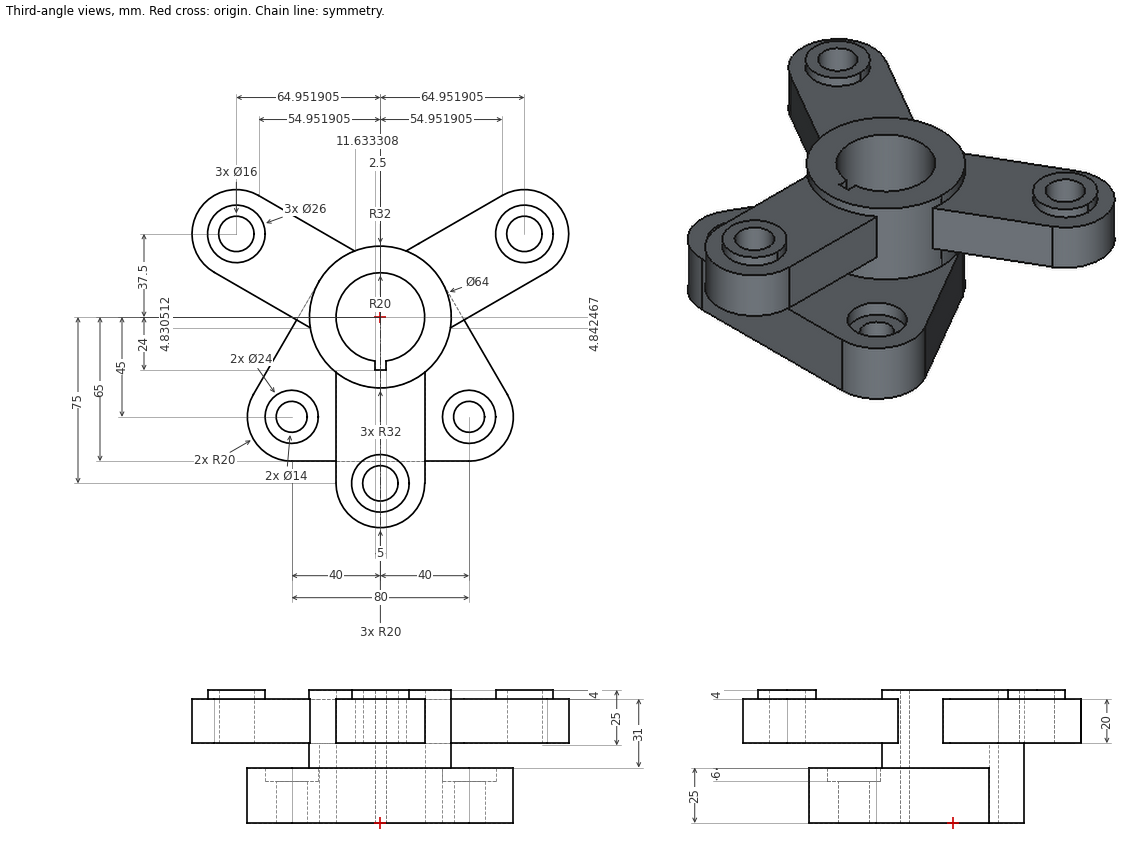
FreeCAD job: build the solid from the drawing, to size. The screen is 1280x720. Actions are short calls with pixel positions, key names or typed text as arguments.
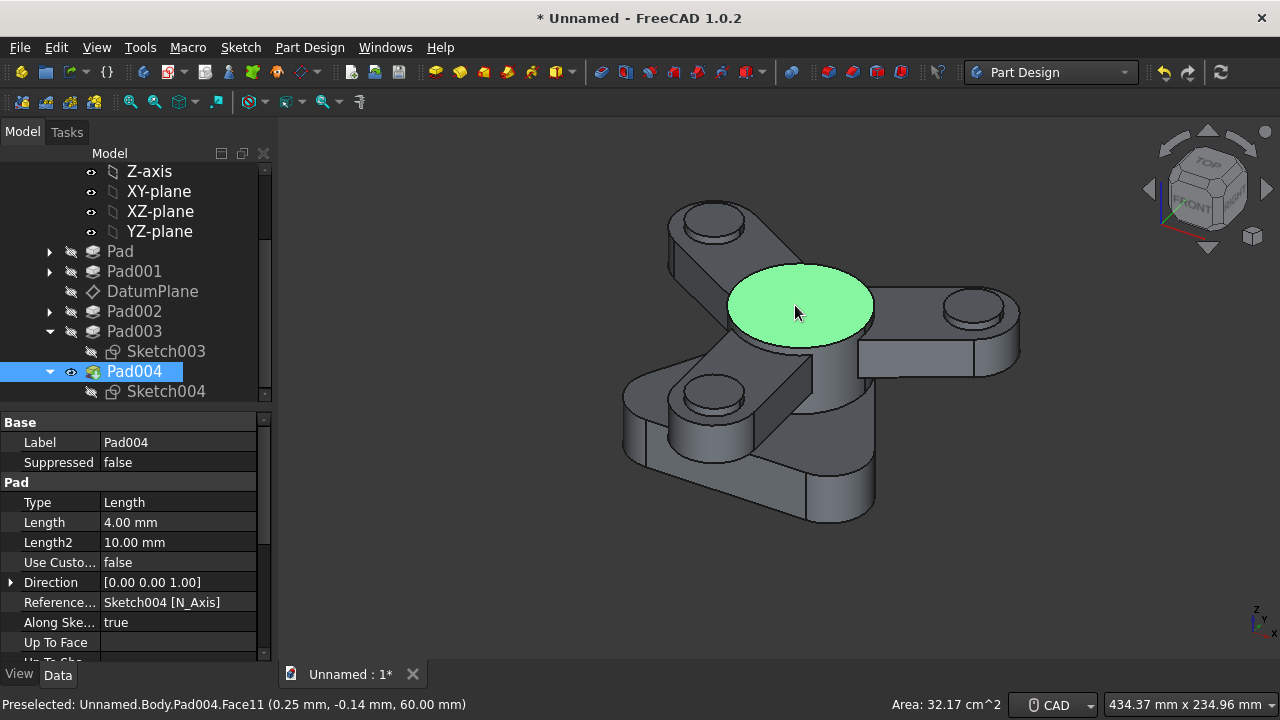
click(168, 72)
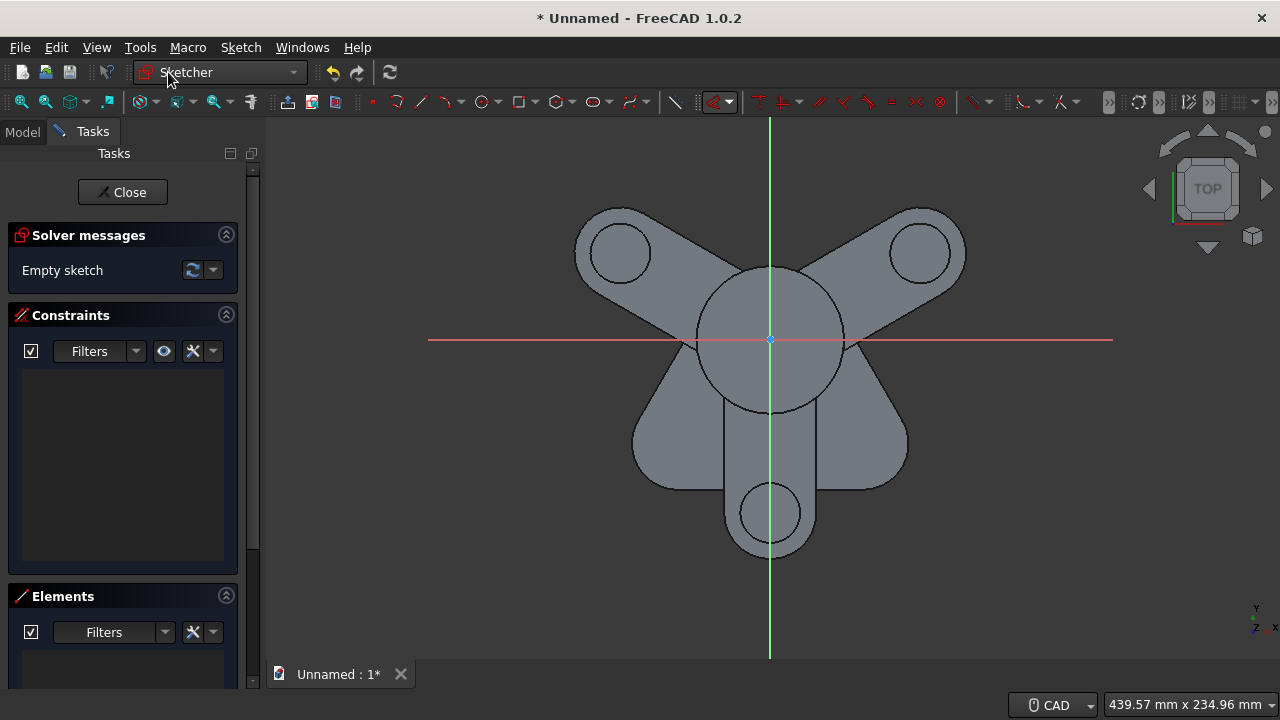
key(g)
key(c)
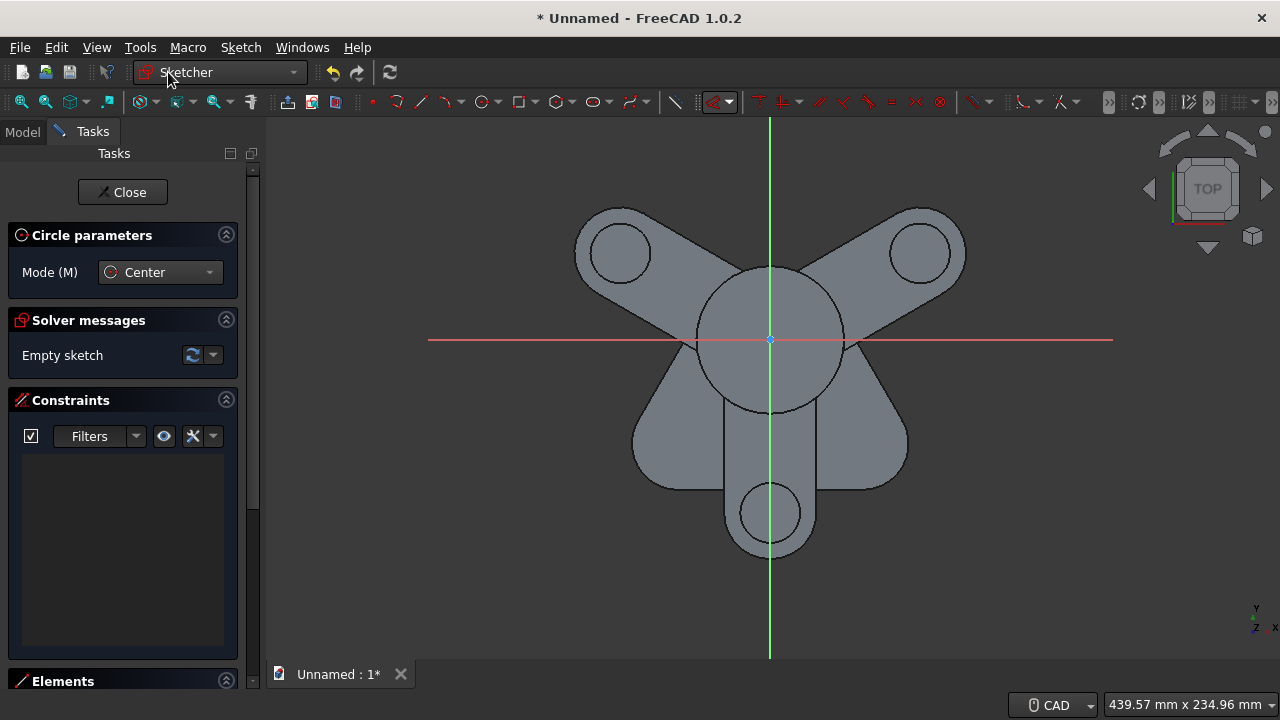
scroll(620, 253, up, 2)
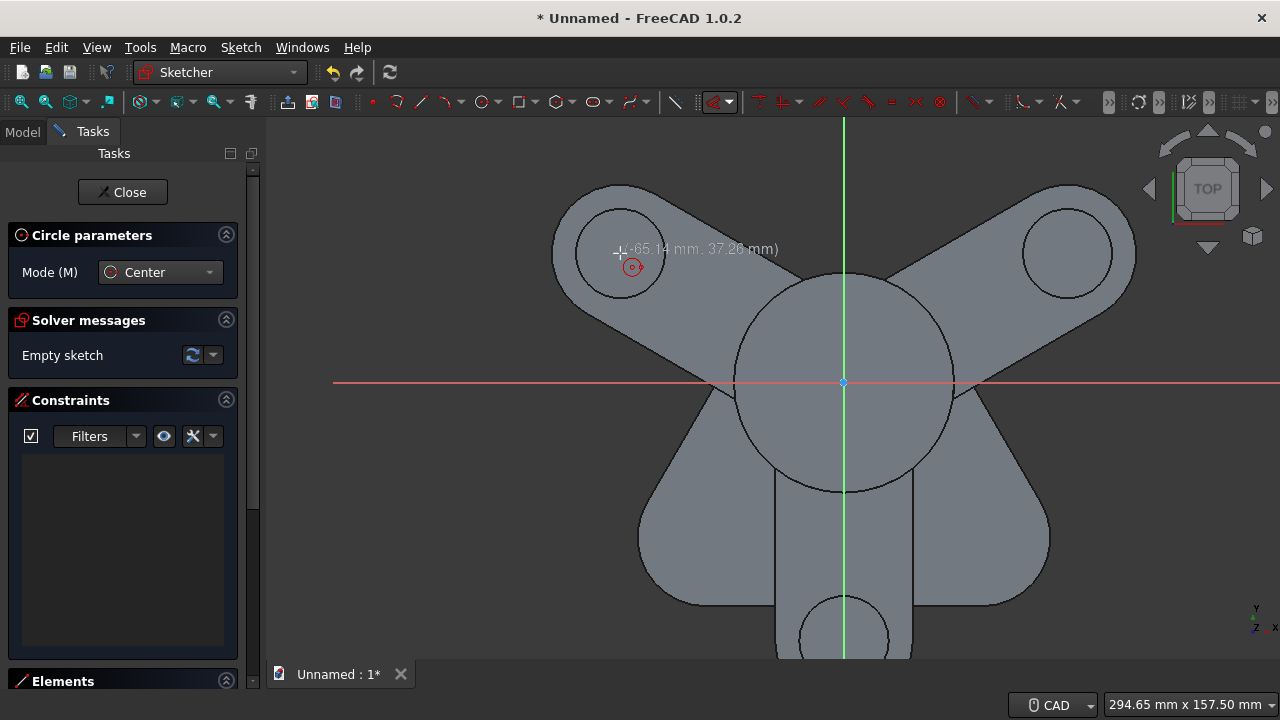
click(620, 254)
click(640, 234)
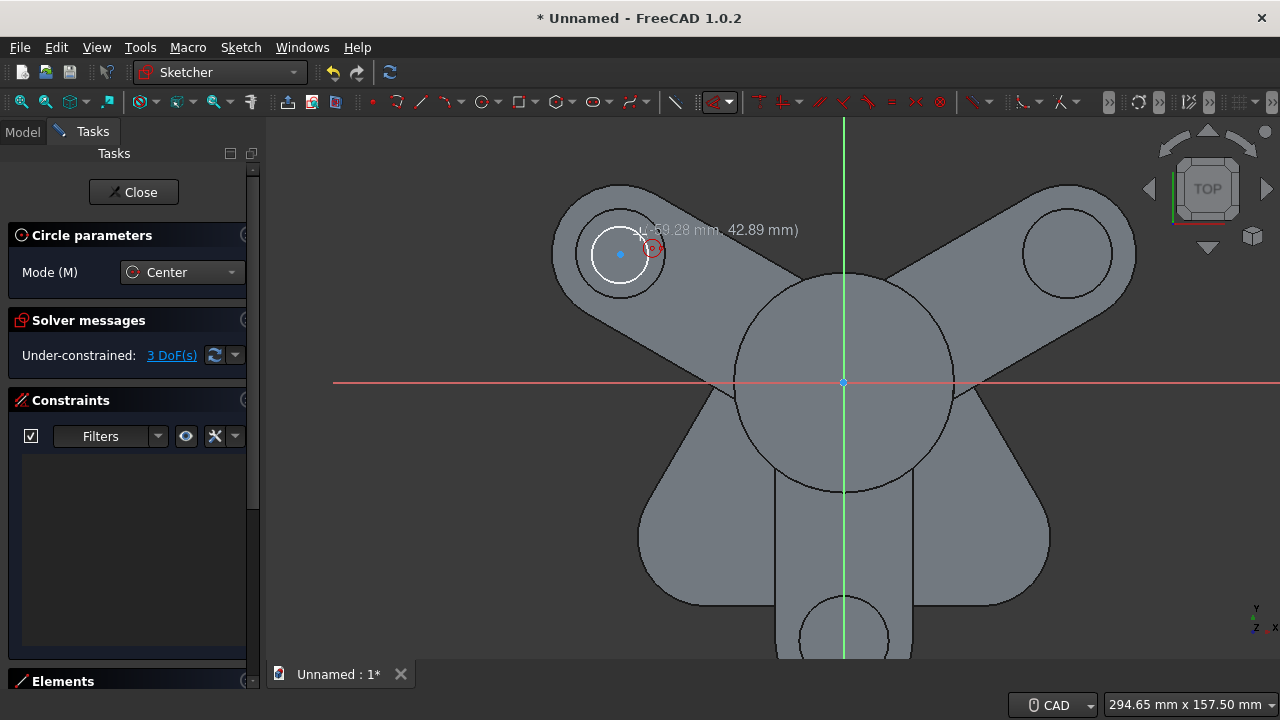
click(1068, 254)
click(1087, 234)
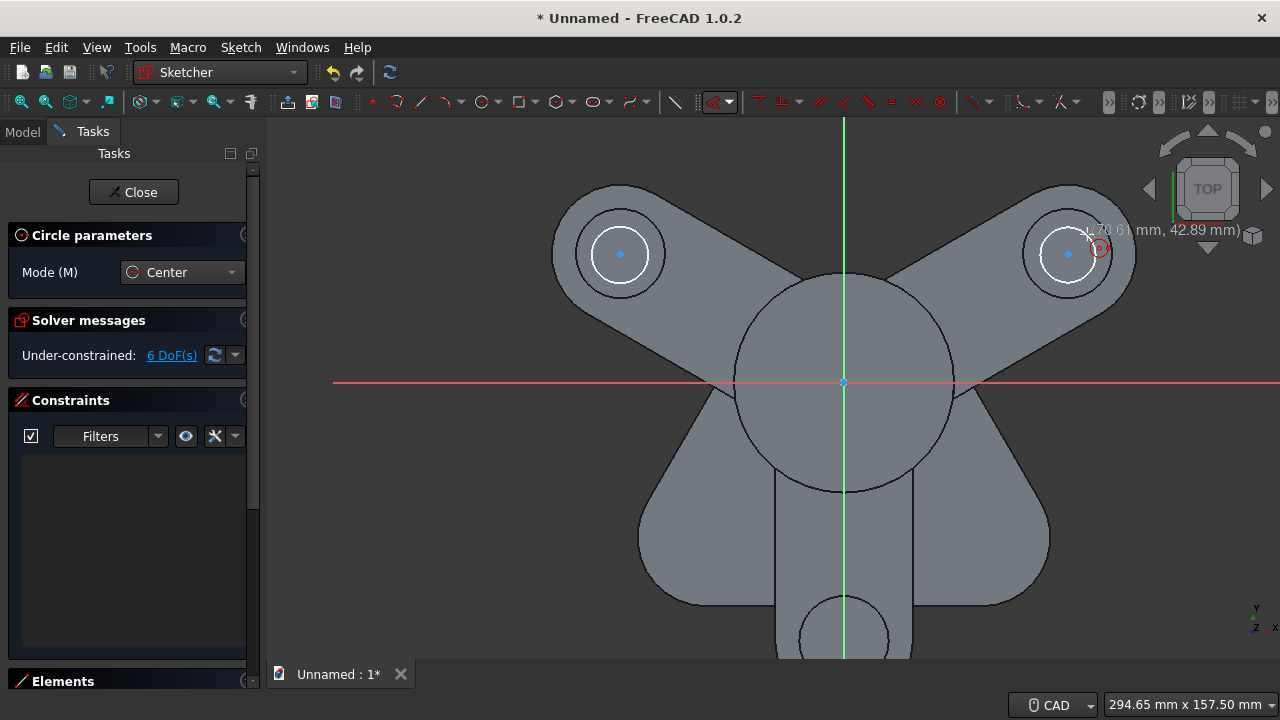
scroll(294, 145, down, 1)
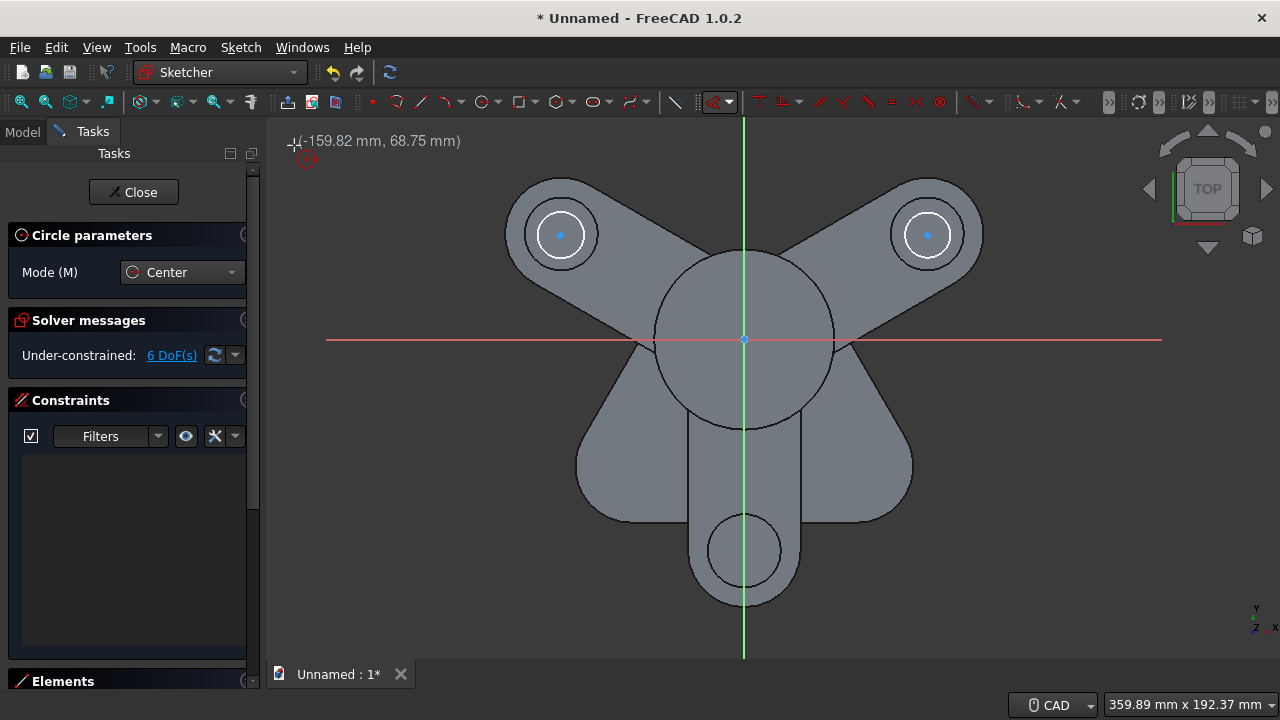
click(744, 551)
click(760, 535)
key(Escape)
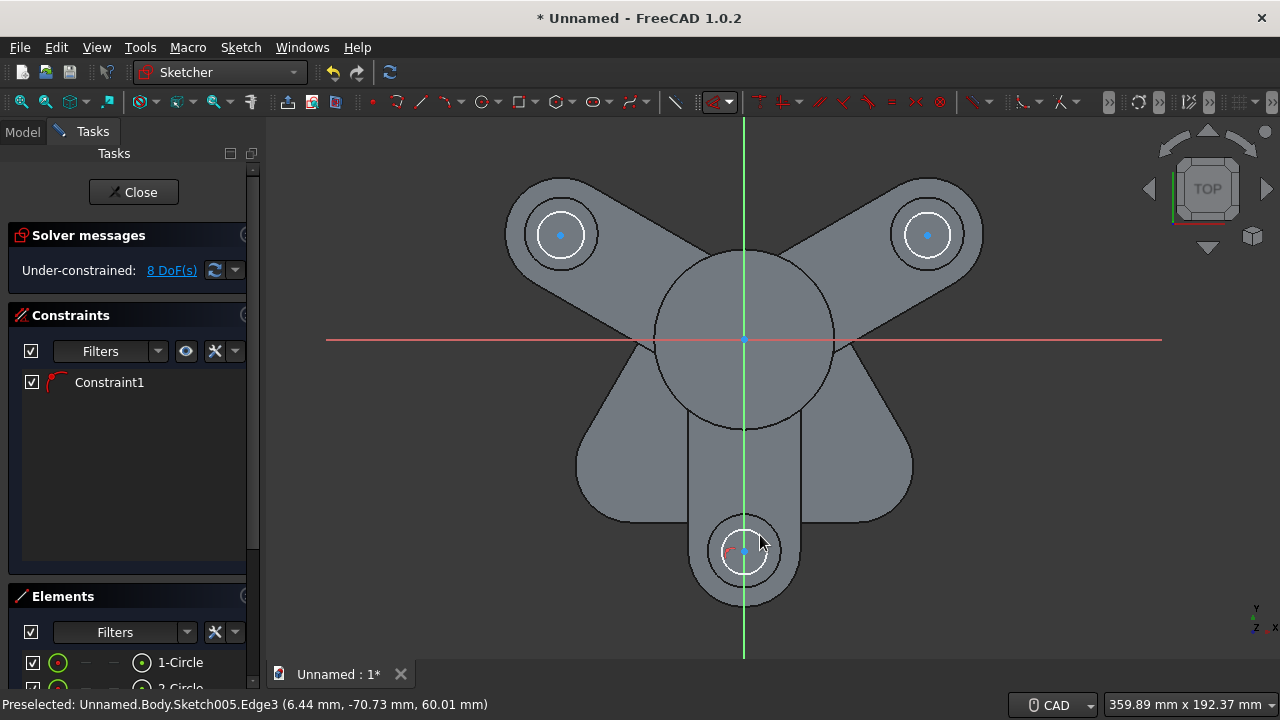
click(577, 219)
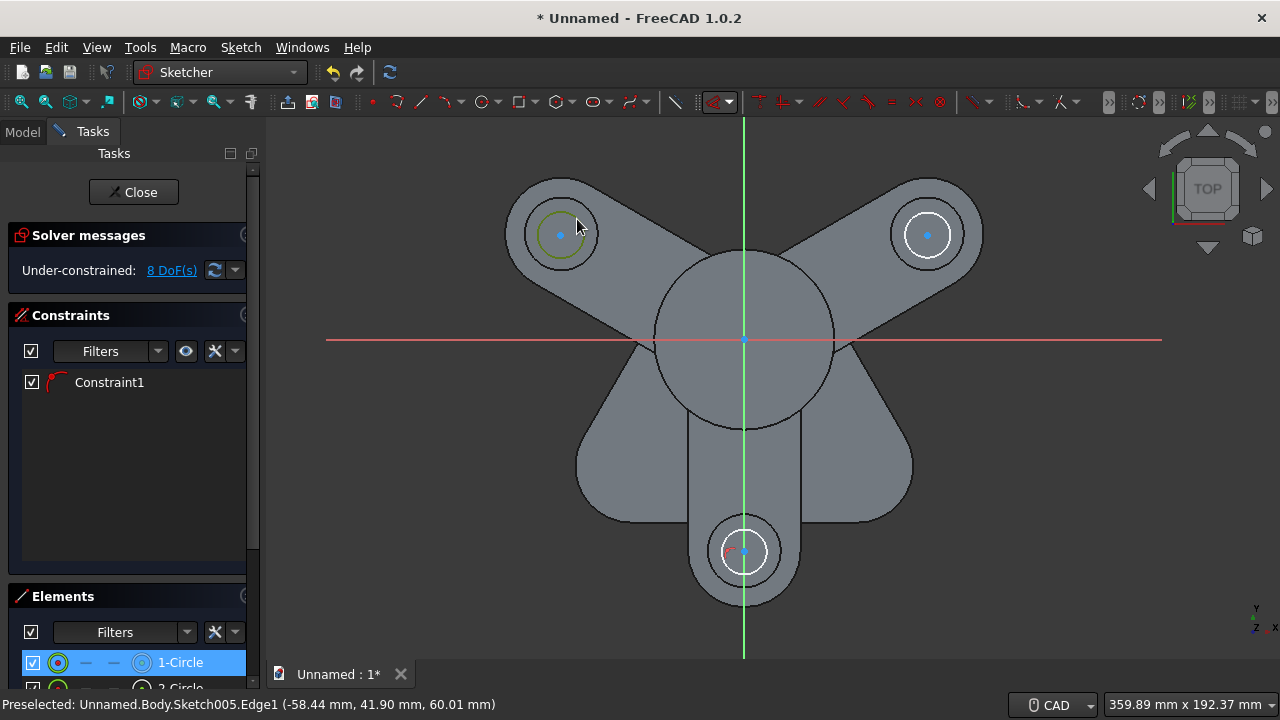
click(944, 219)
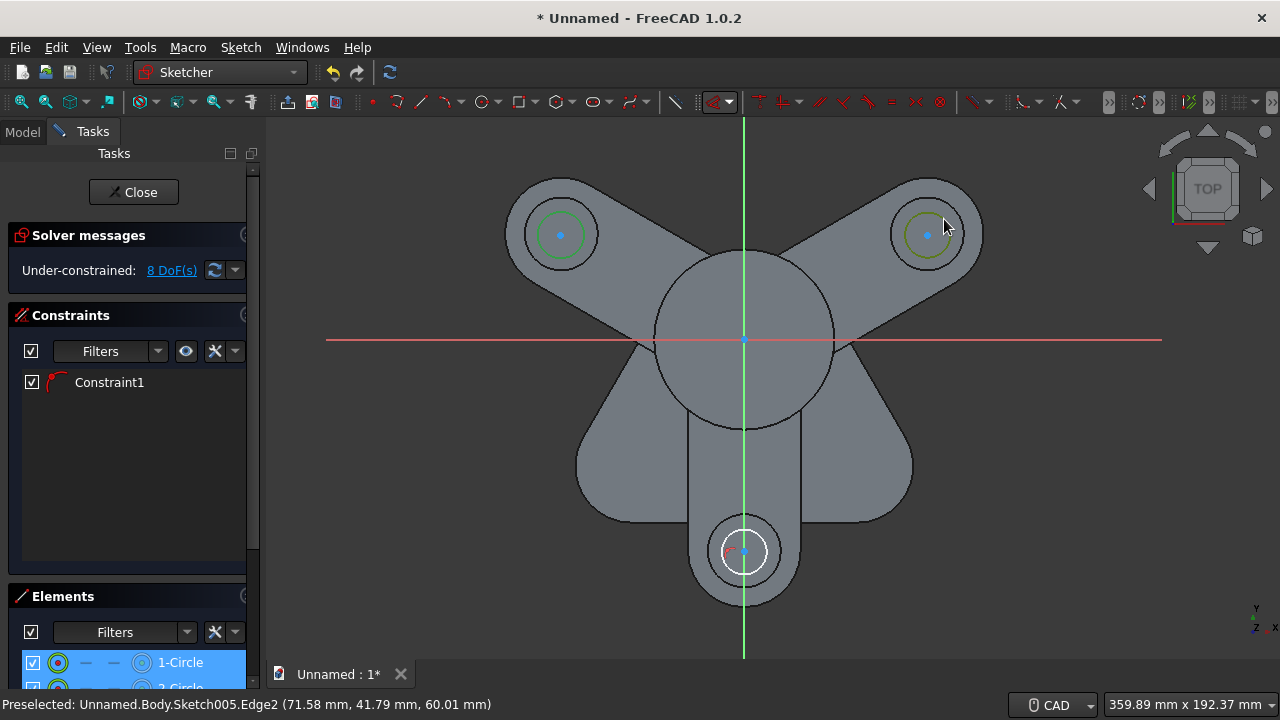
click(760, 536)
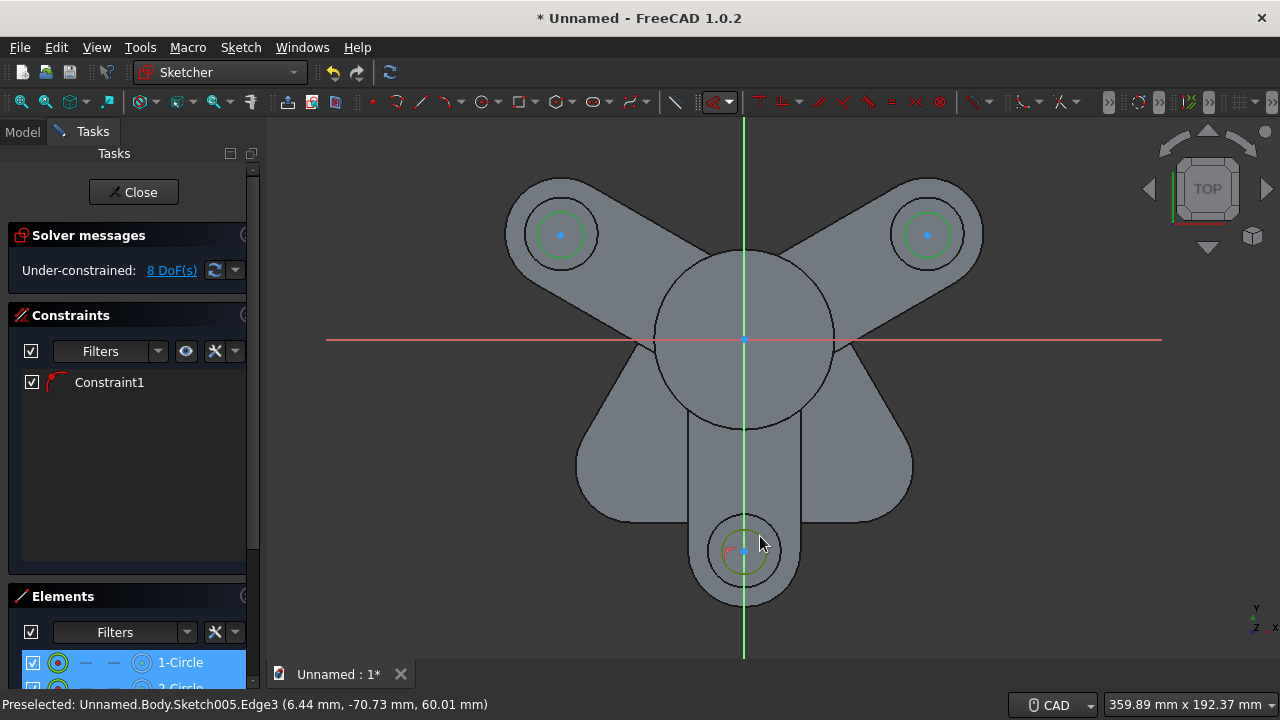
key(e)